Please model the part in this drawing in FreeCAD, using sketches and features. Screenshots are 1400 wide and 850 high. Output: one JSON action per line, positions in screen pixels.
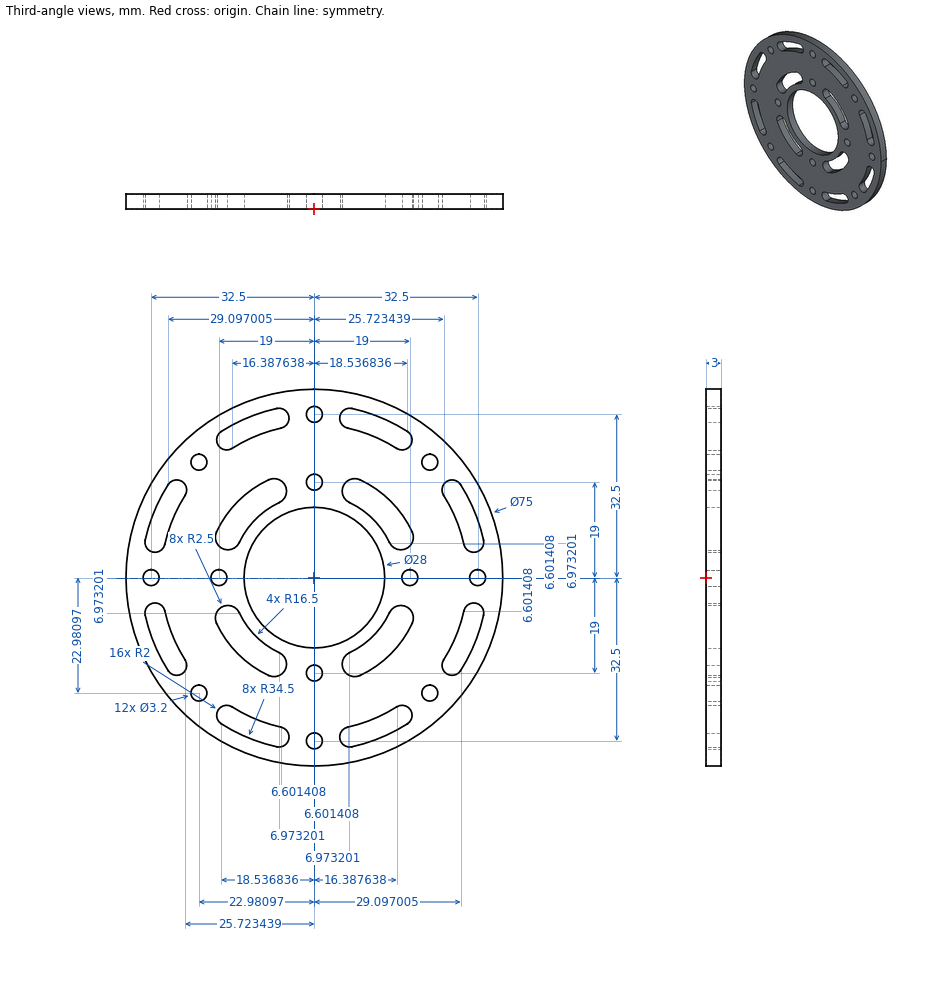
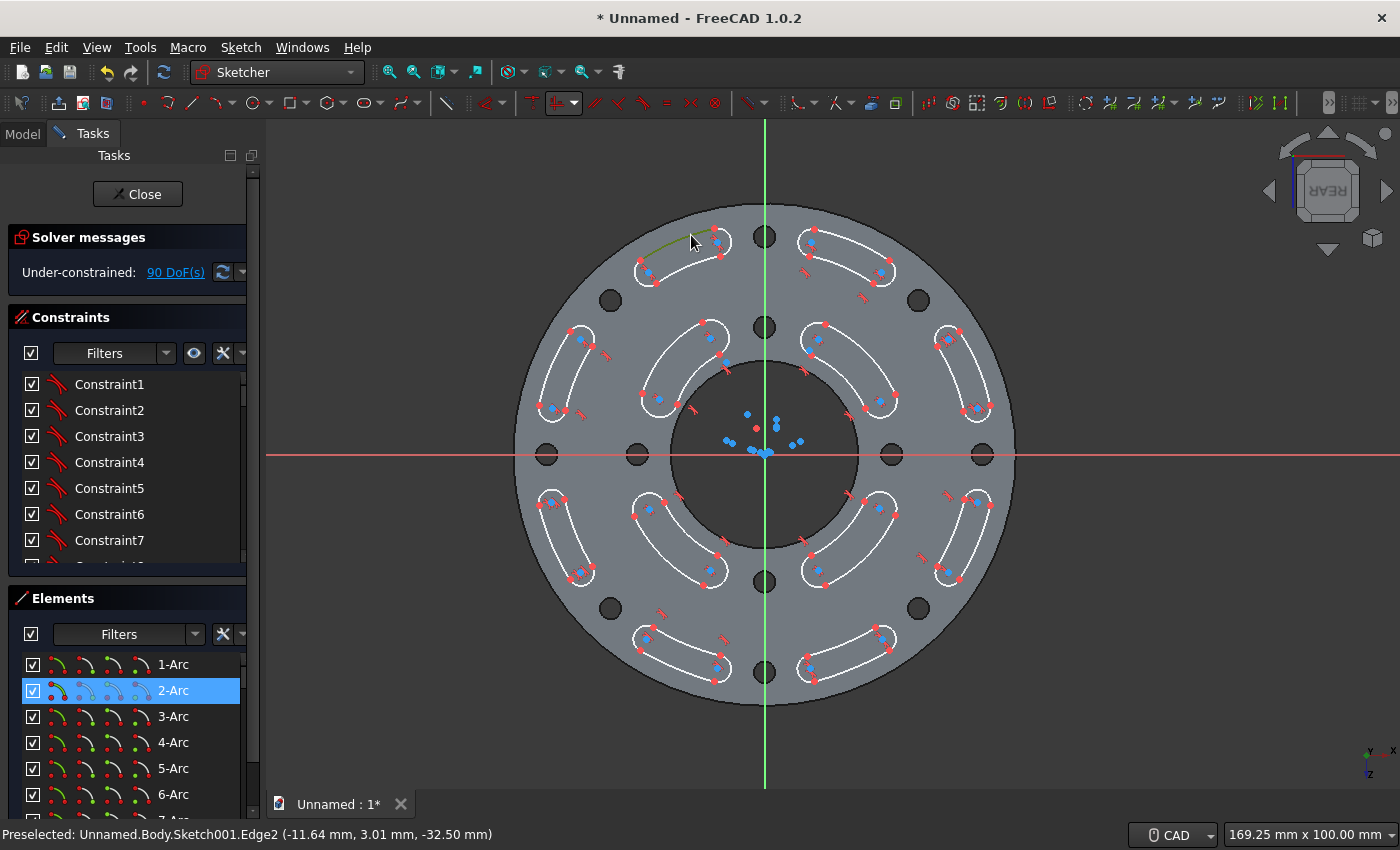
{"action": "left_click", "coordinate": [855, 273]}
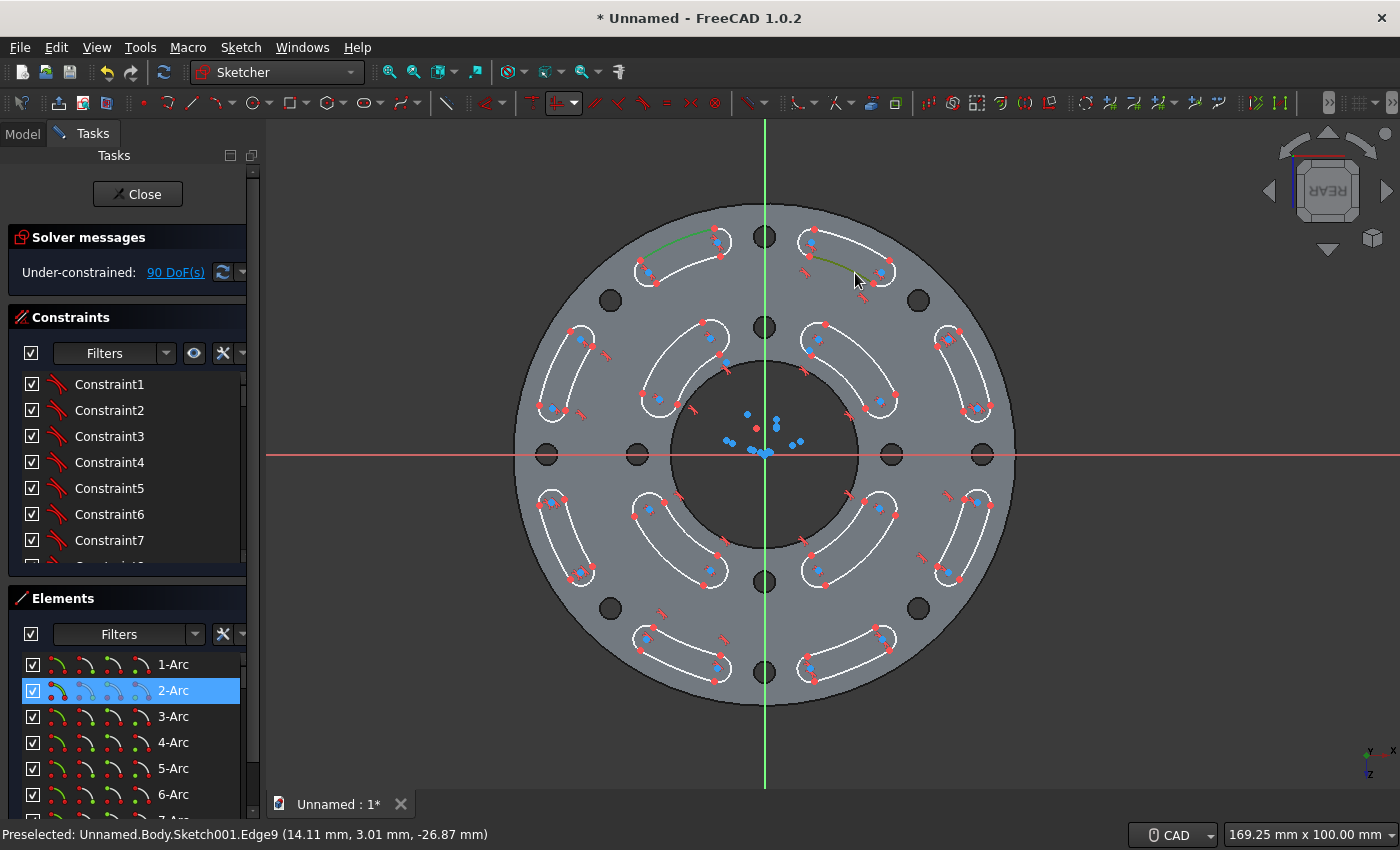
{"action": "left_click", "coordinate": [532, 104]}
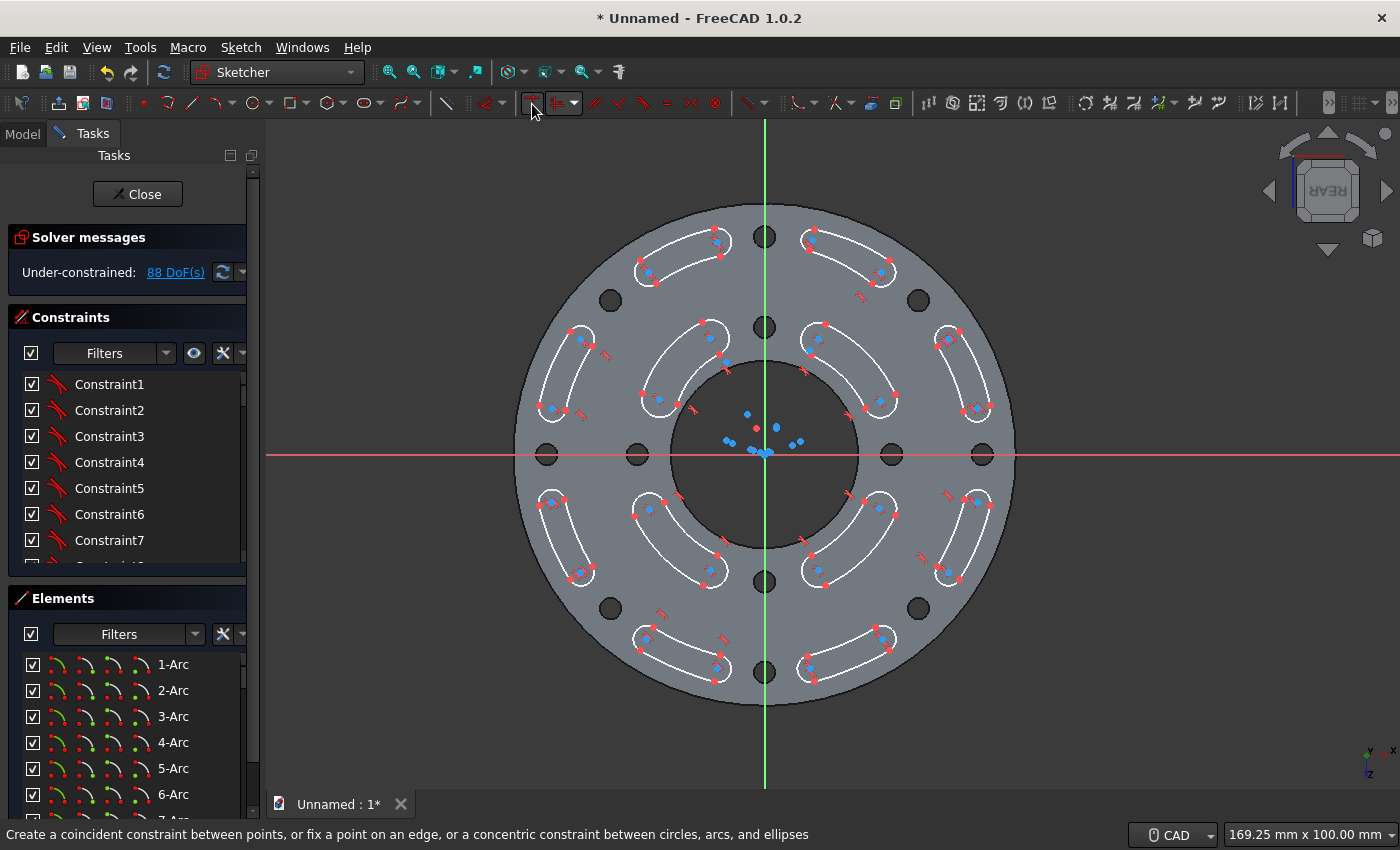
{"action": "left_click", "coordinate": [691, 235]}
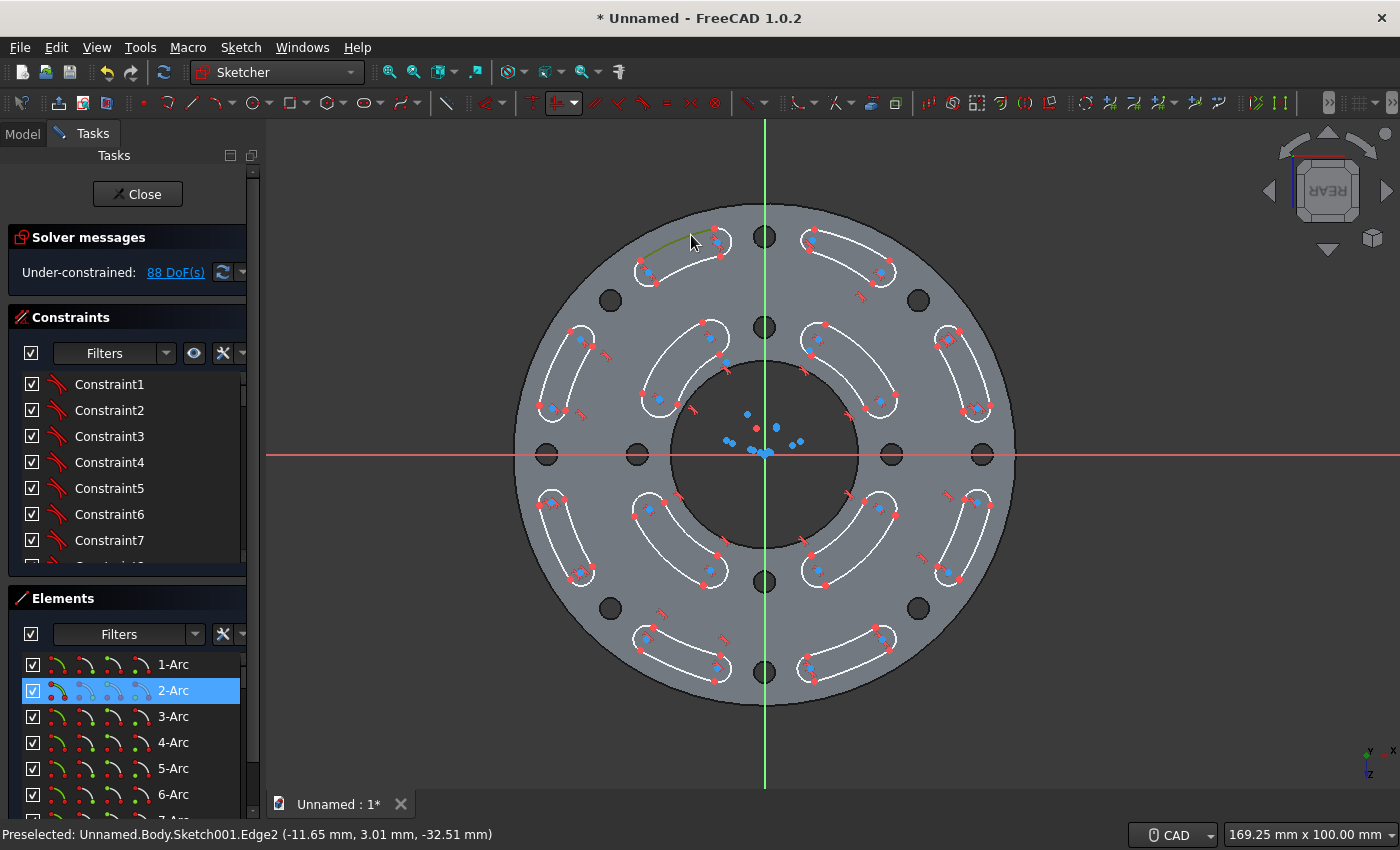
{"action": "left_click", "coordinate": [868, 248]}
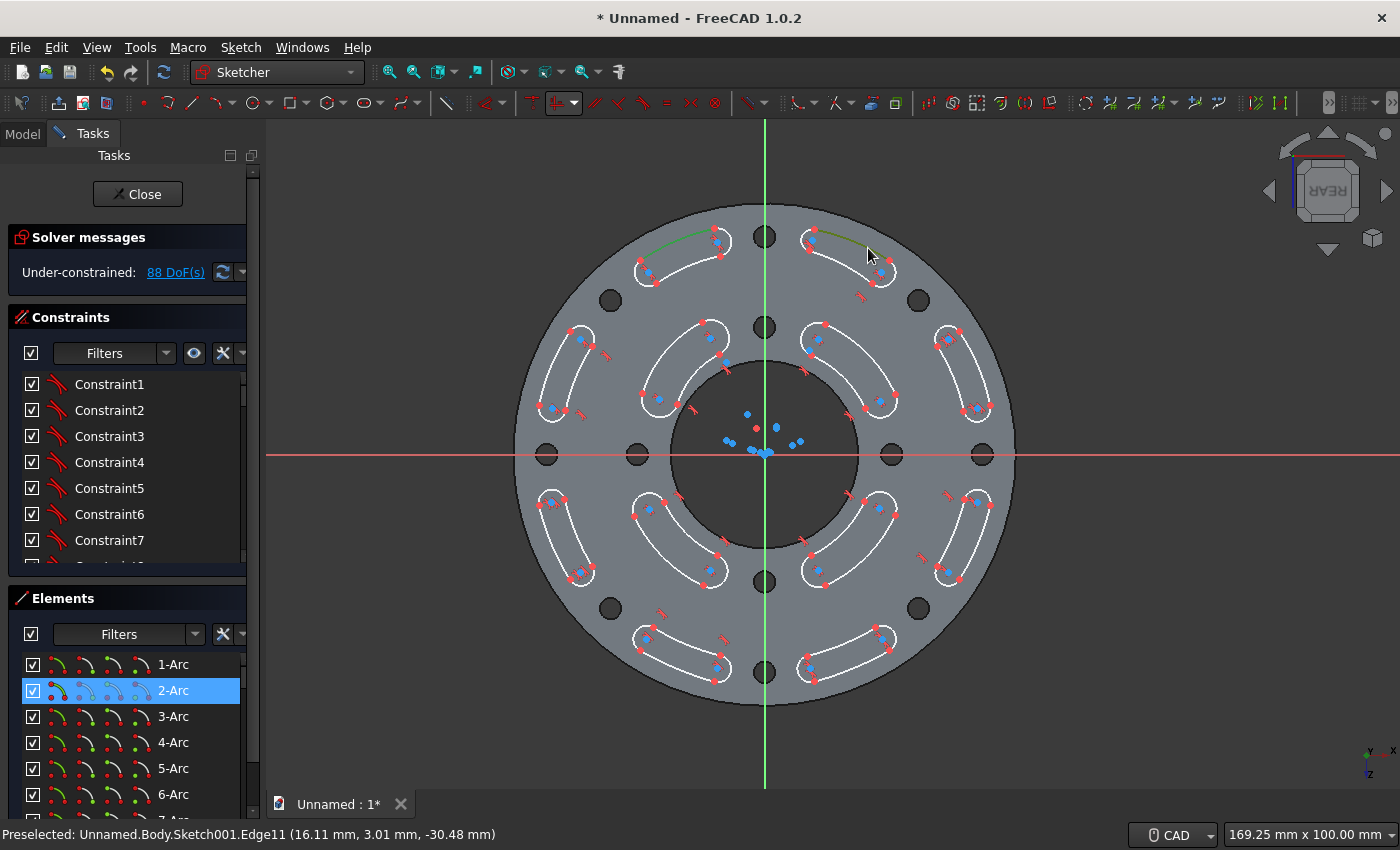
{"action": "left_click", "coordinate": [532, 104]}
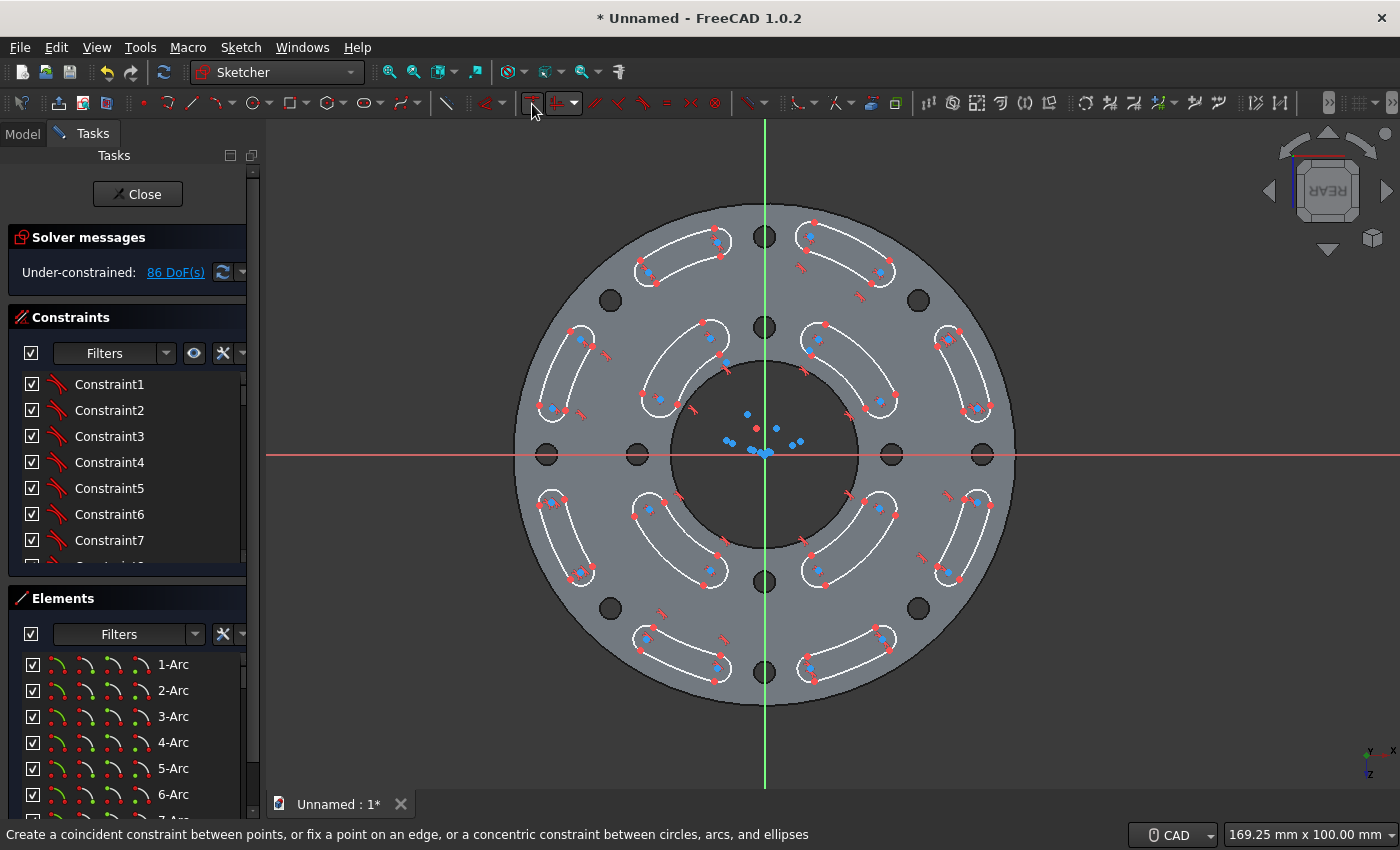
{"action": "left_click", "coordinate": [691, 235]}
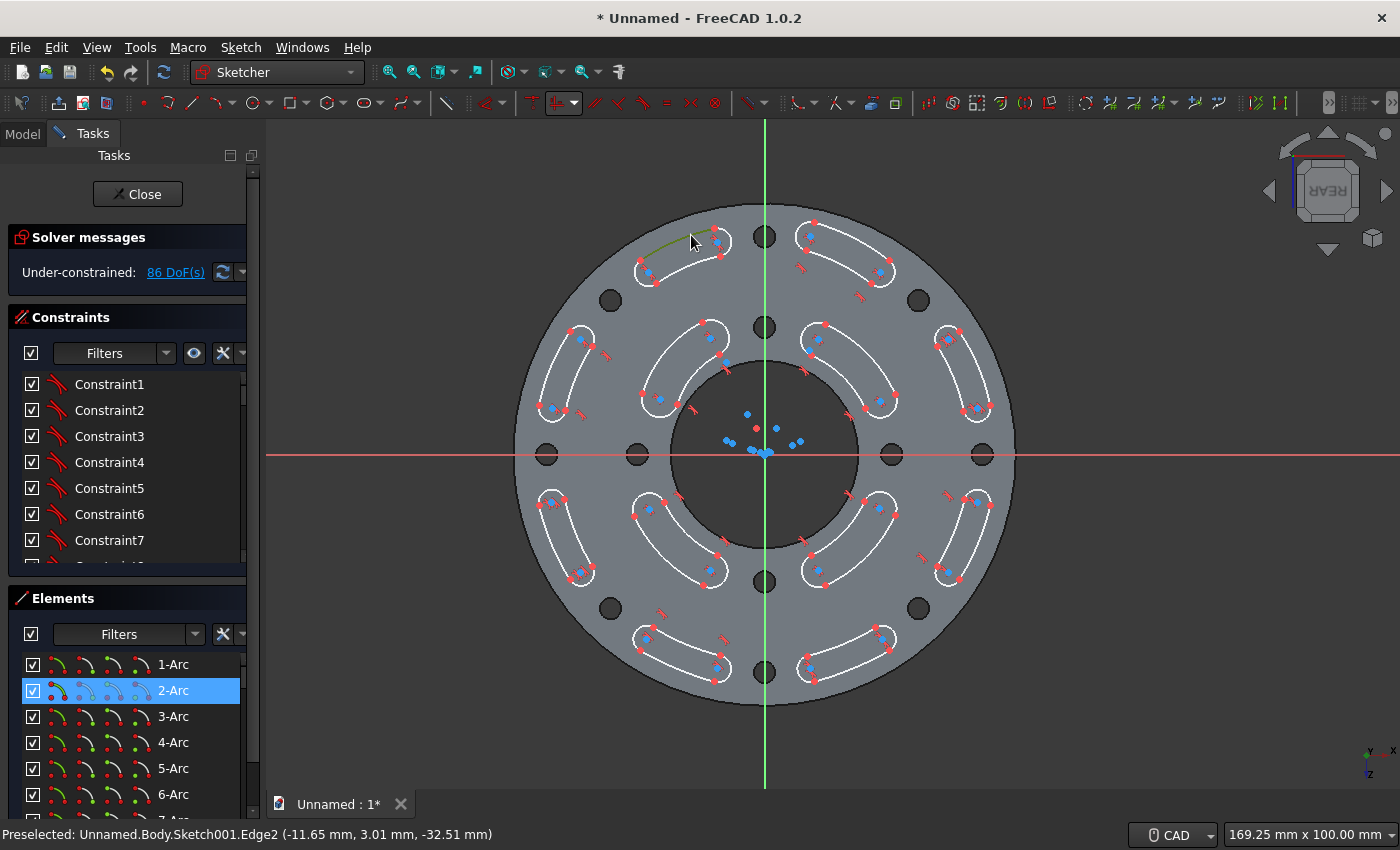
{"action": "left_click", "coordinate": [984, 382]}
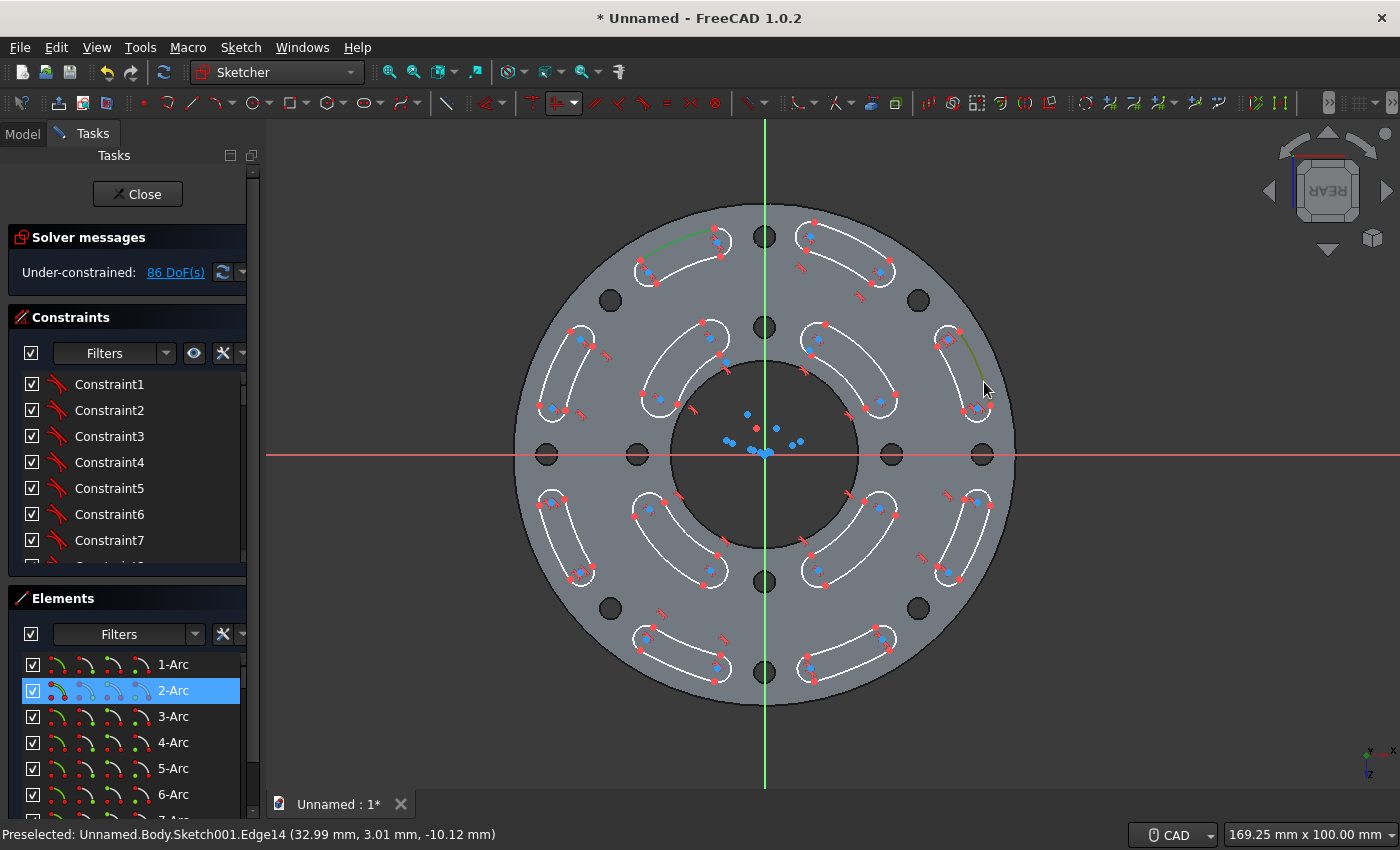
{"action": "left_click", "coordinate": [532, 104]}